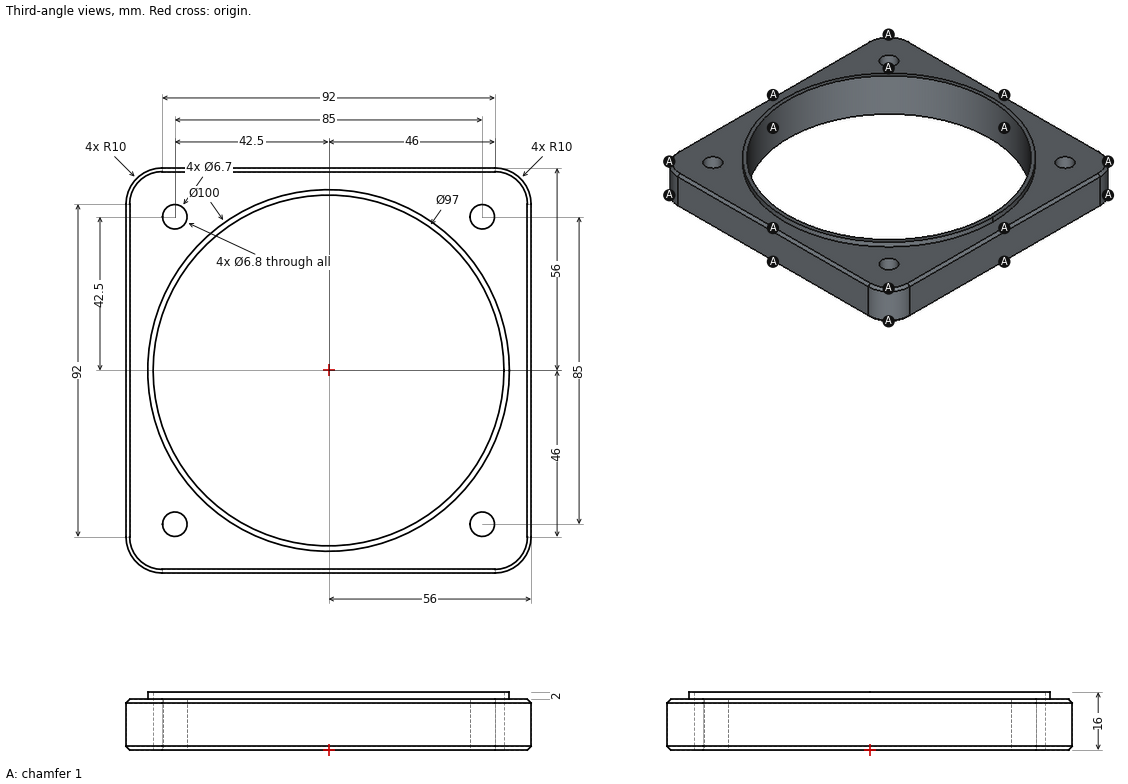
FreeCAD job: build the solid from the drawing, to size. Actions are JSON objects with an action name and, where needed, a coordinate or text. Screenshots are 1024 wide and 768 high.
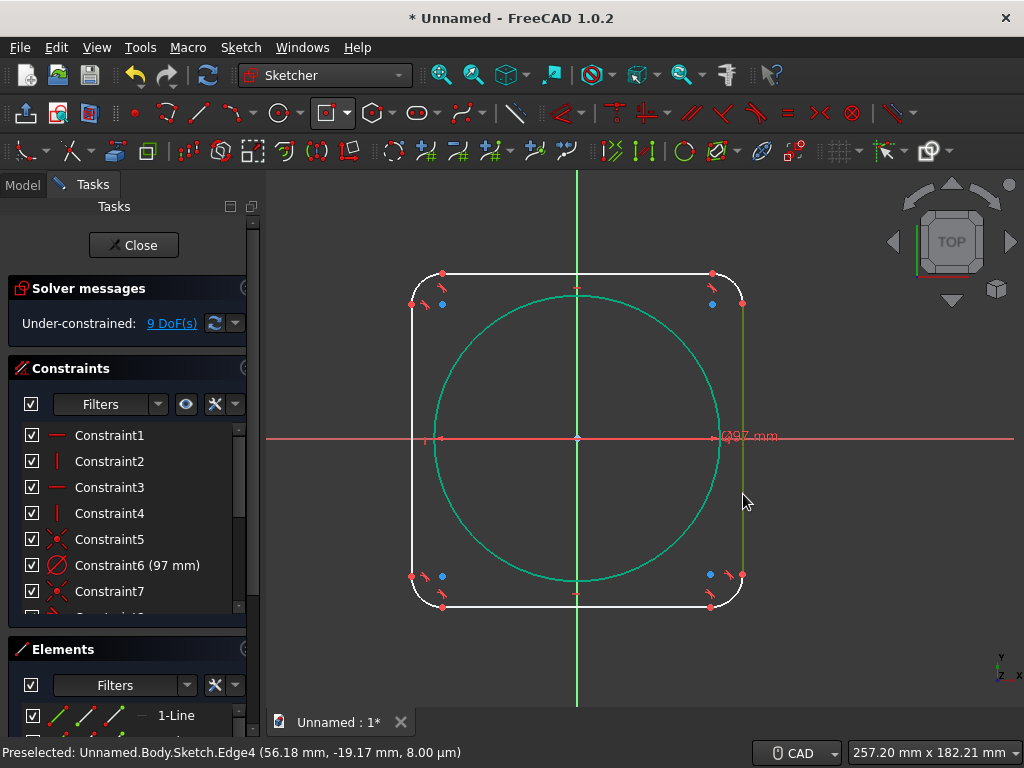
{"action": "left_click", "coordinate": [739, 290]}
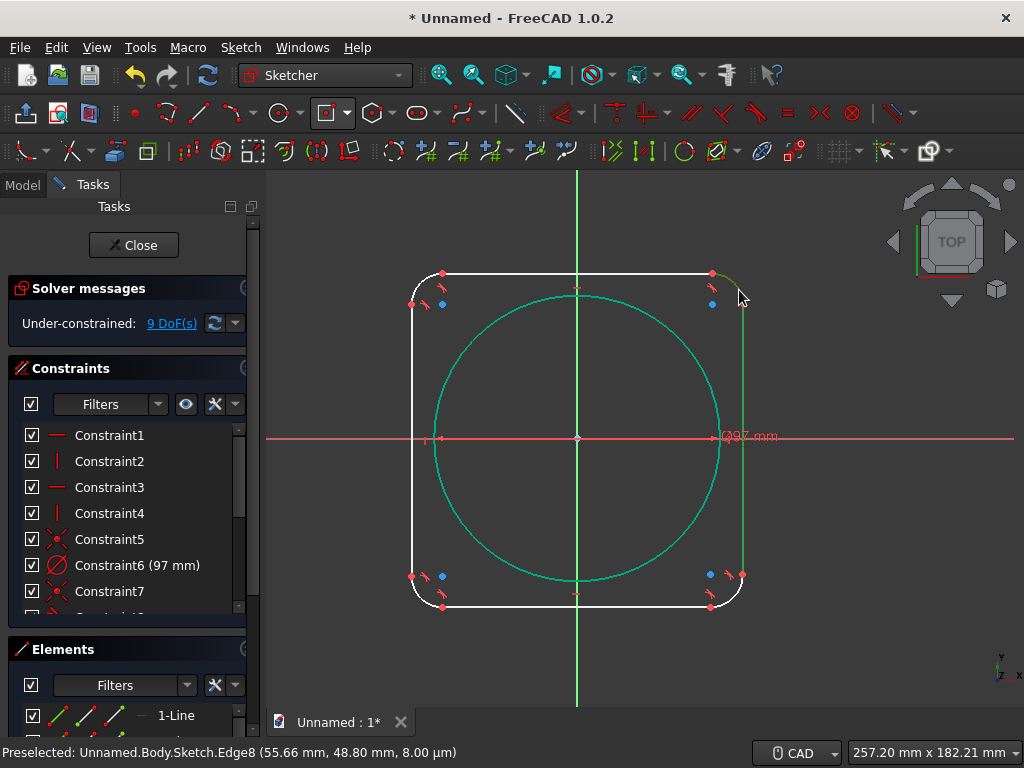
{"action": "left_click", "coordinate": [756, 114]}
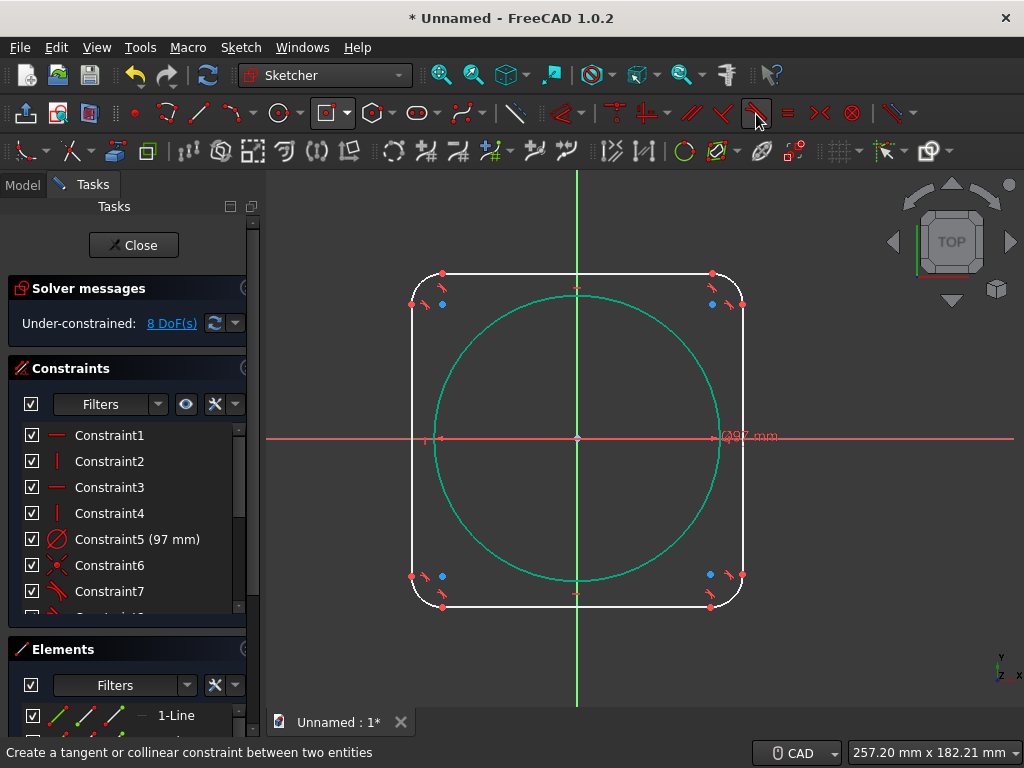
{"action": "left_click", "coordinate": [429, 277]}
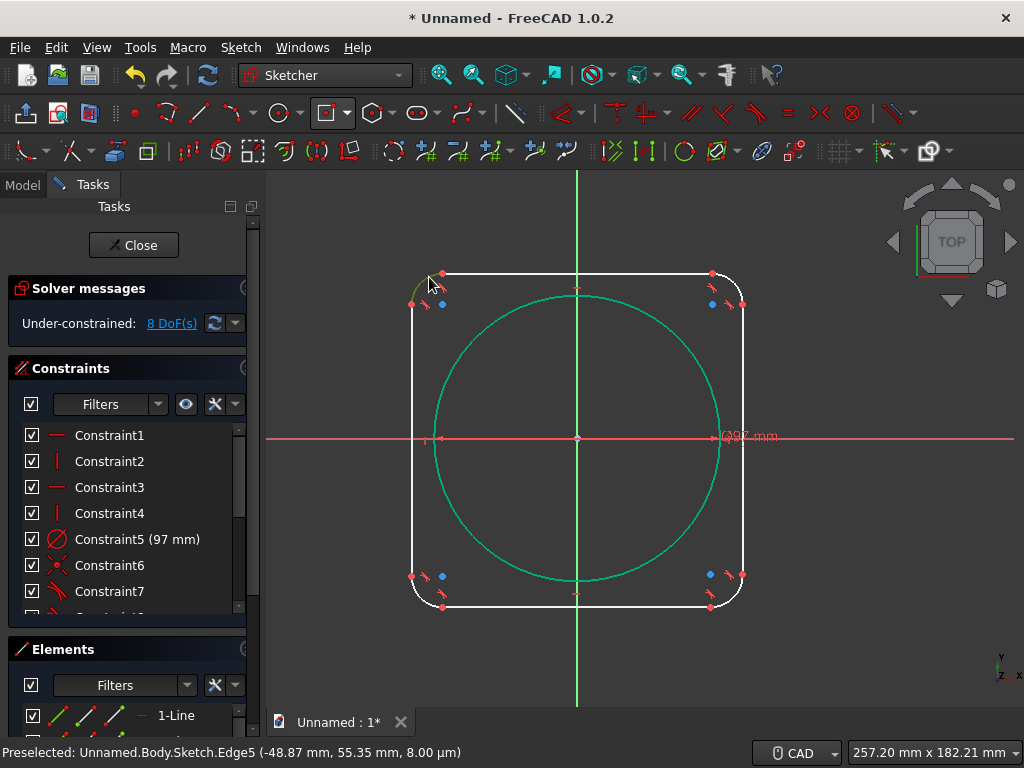
{"action": "left_click", "coordinate": [415, 591]}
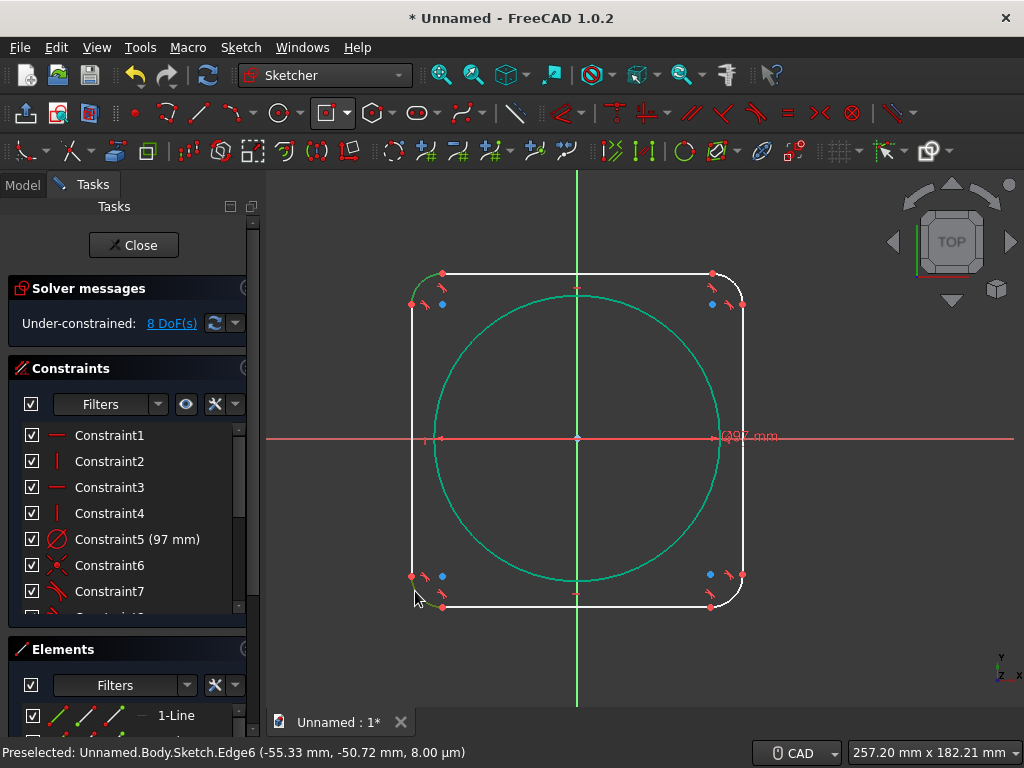
{"action": "left_click", "coordinate": [725, 604]}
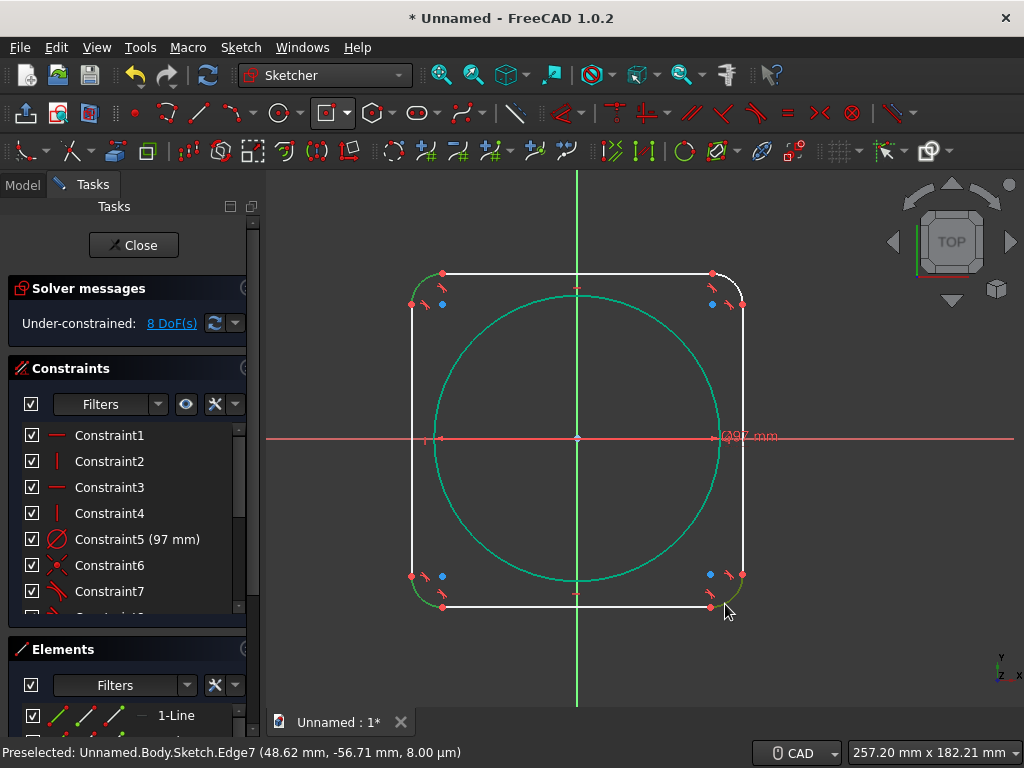
{"action": "left_click", "coordinate": [739, 290]}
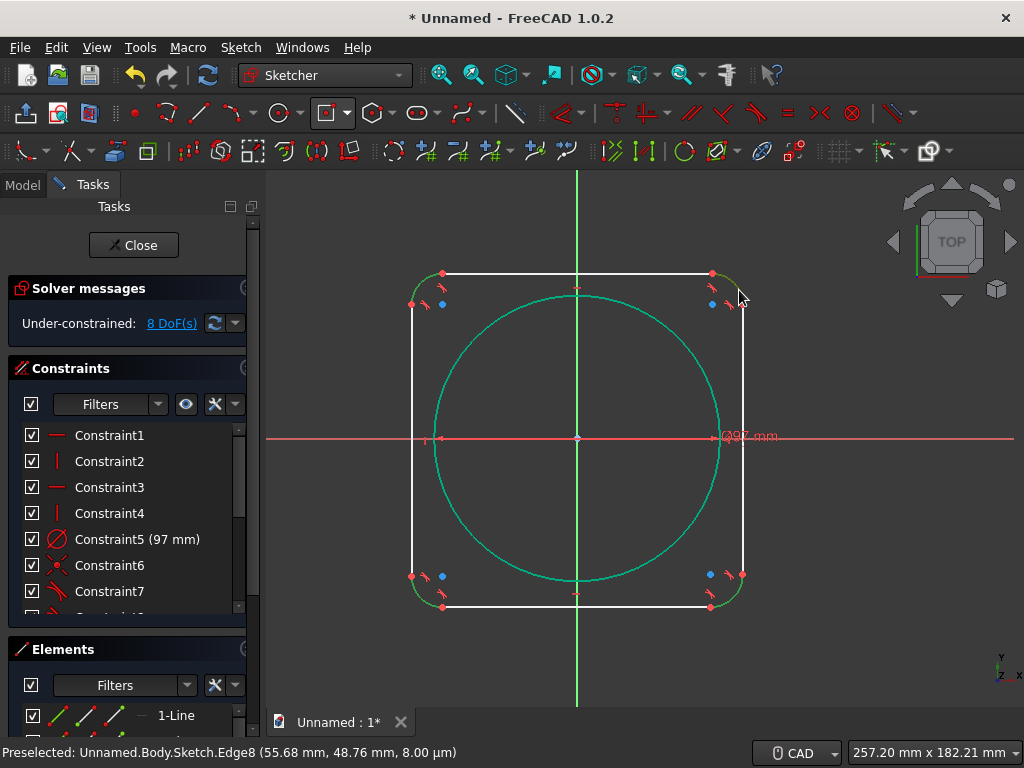
{"action": "left_click", "coordinate": [788, 114]}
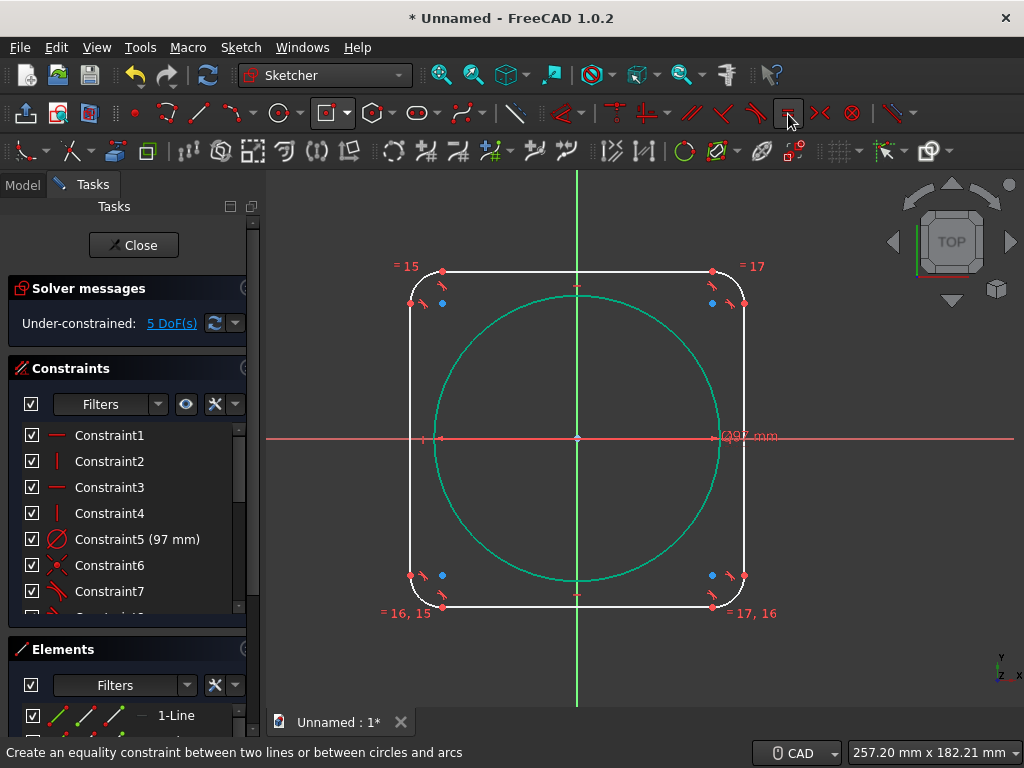
{"action": "left_click", "coordinate": [562, 114]}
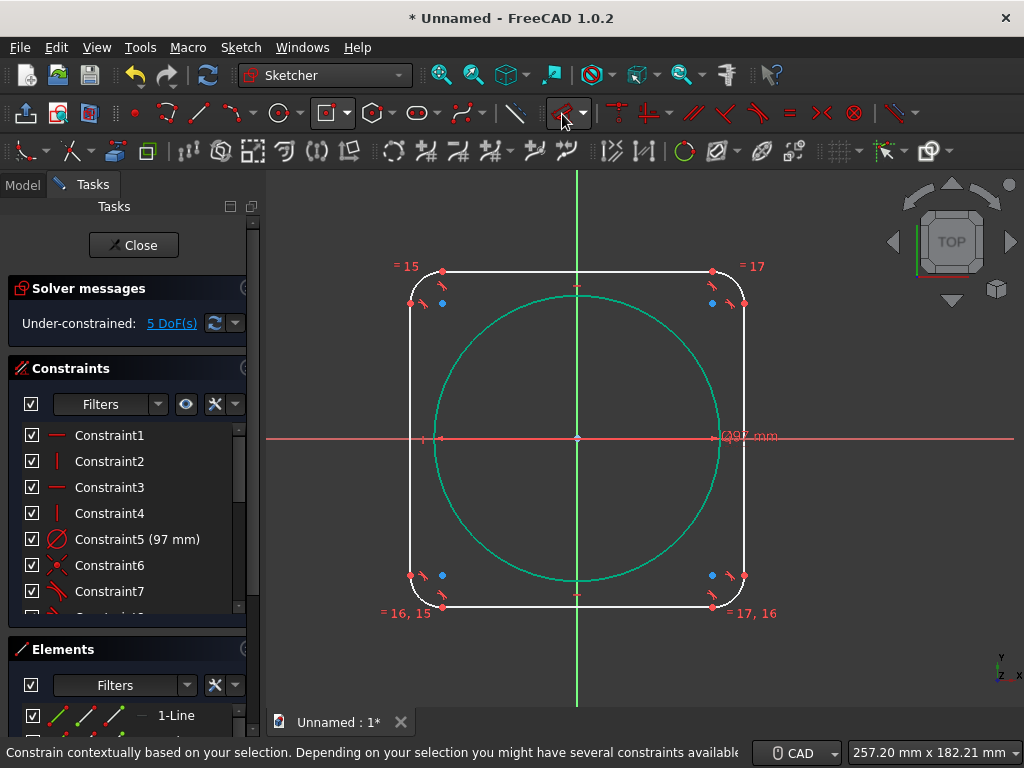
{"action": "scroll", "coordinate": [428, 275], "scroll_direction": "up", "scroll_amount": 2}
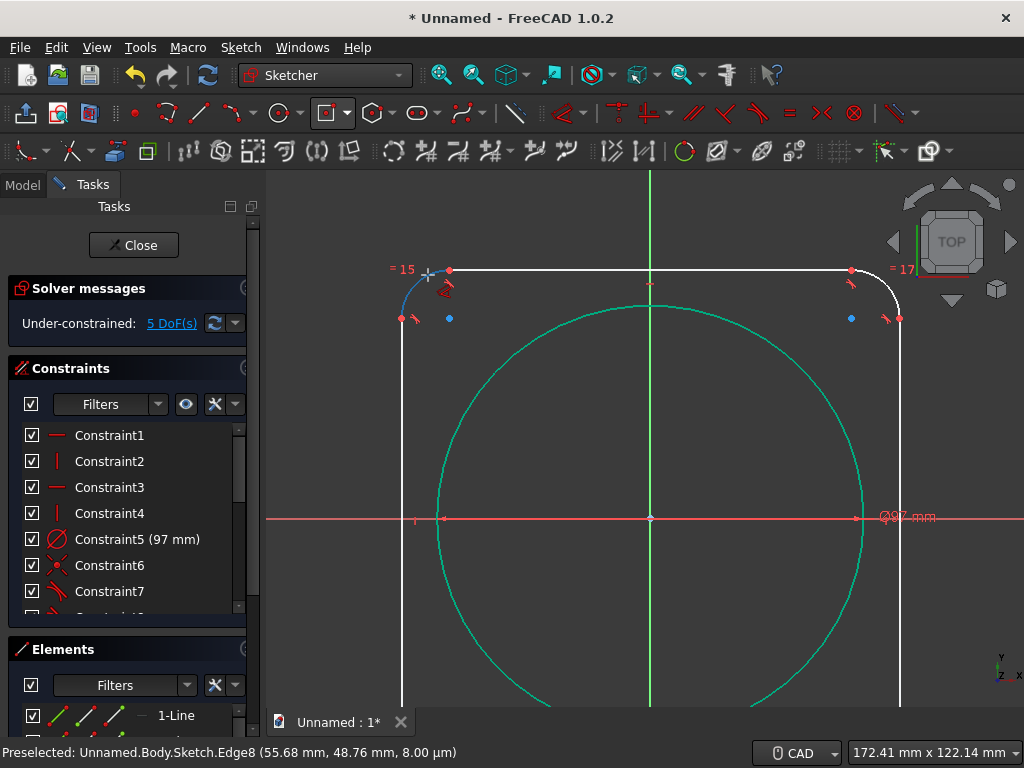
{"action": "left_click", "coordinate": [428, 275]}
{"action": "left_click", "coordinate": [414, 246]}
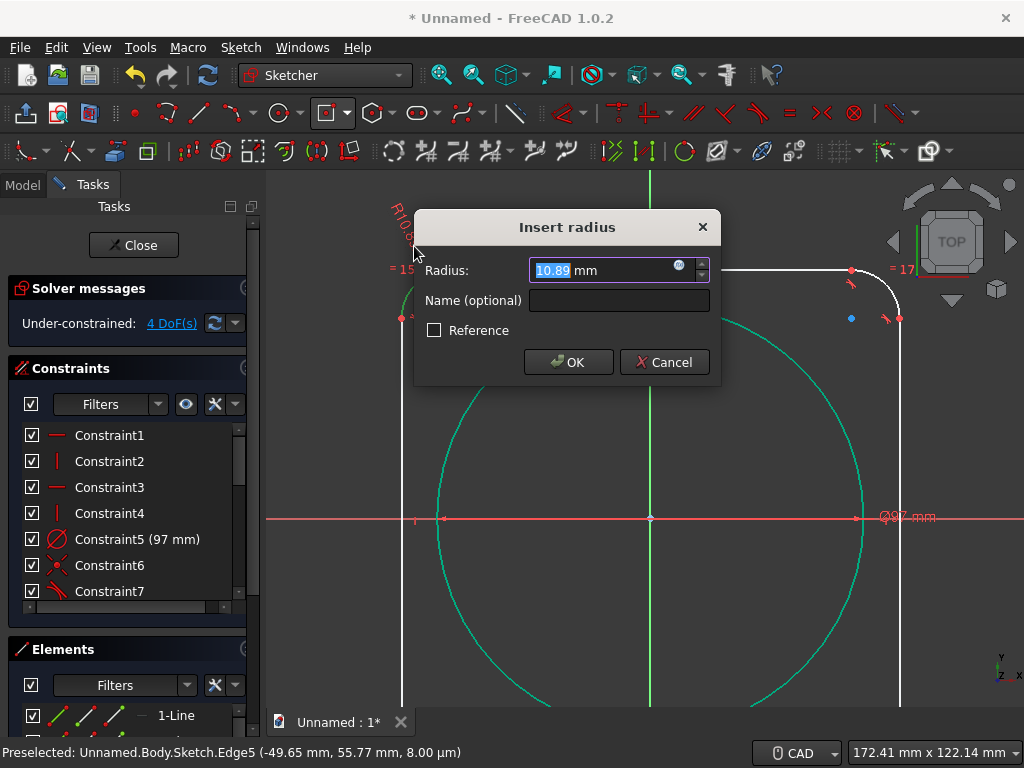
{"action": "type", "text": "10"}
{"action": "key", "text": "Return"}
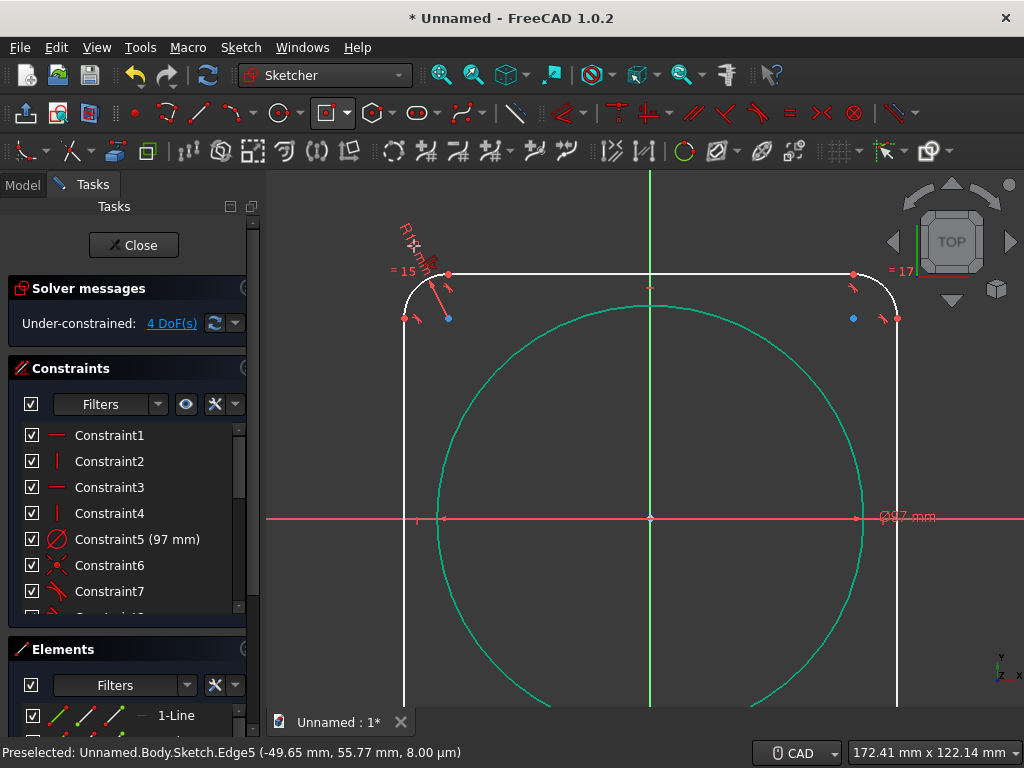
{"action": "left_click", "coordinate": [732, 274]}
{"action": "left_click", "coordinate": [558, 240]}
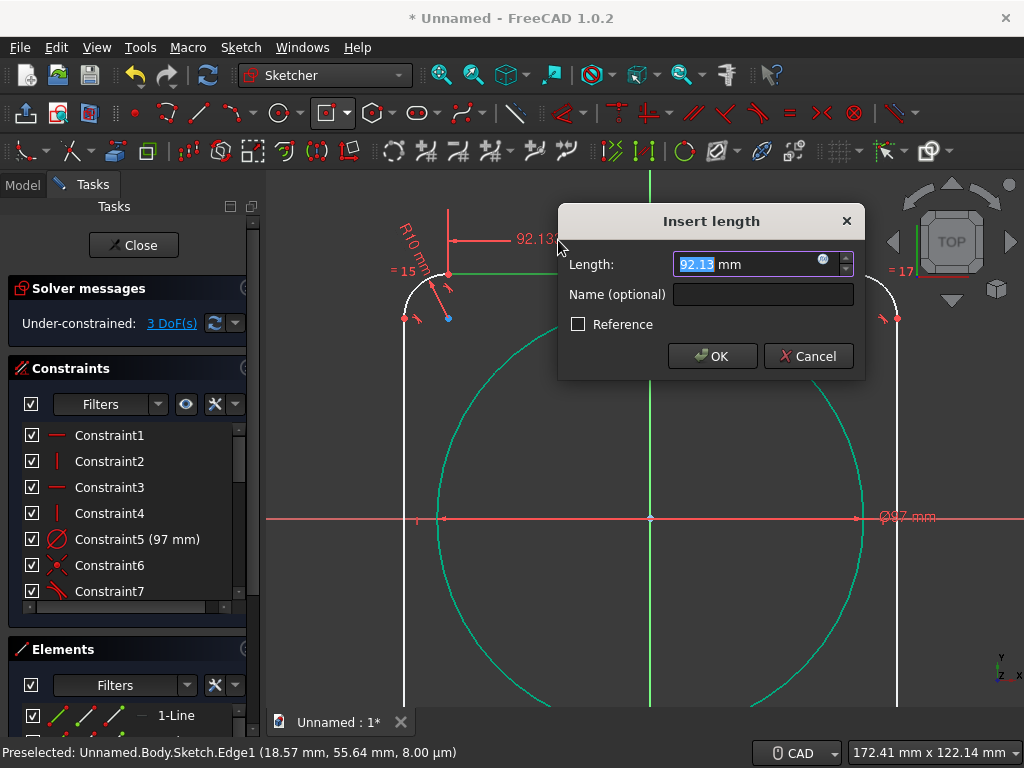
{"action": "type", "text": "92"}
{"action": "key", "text": "Return"}